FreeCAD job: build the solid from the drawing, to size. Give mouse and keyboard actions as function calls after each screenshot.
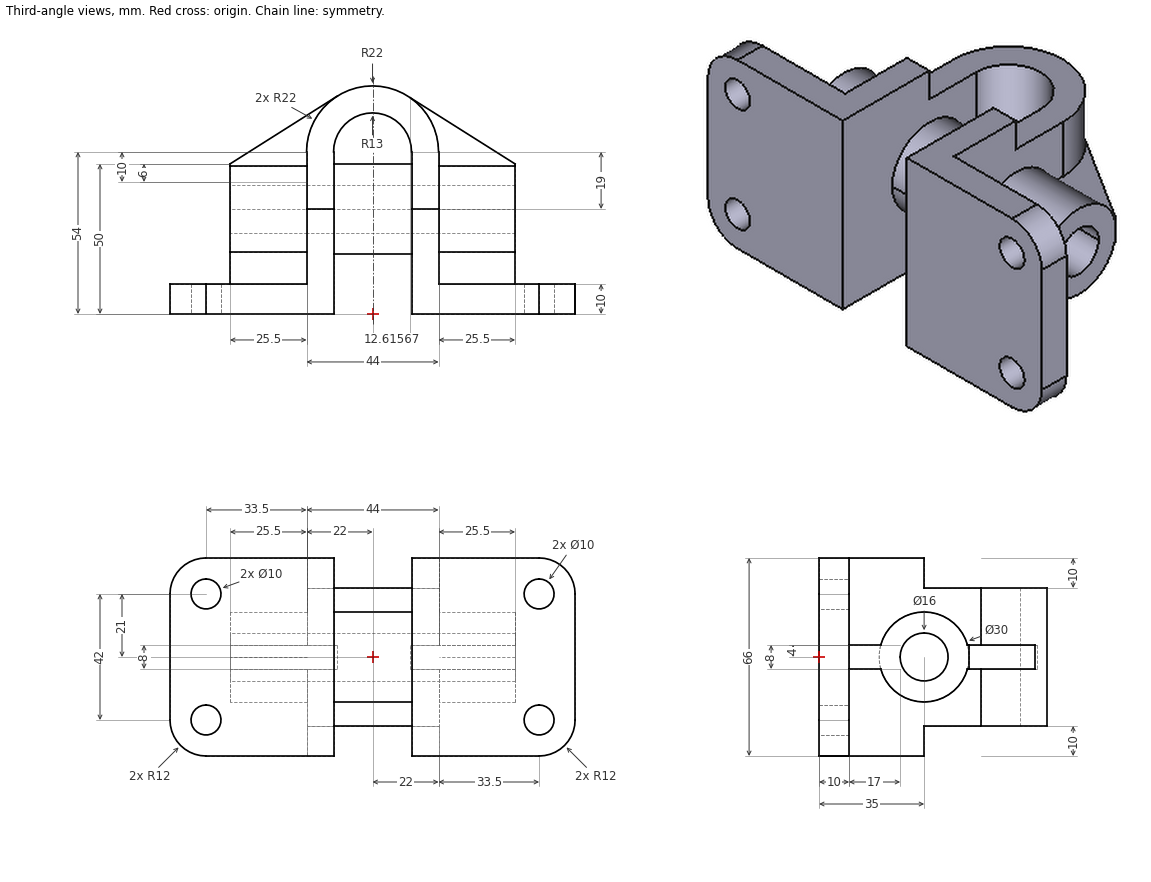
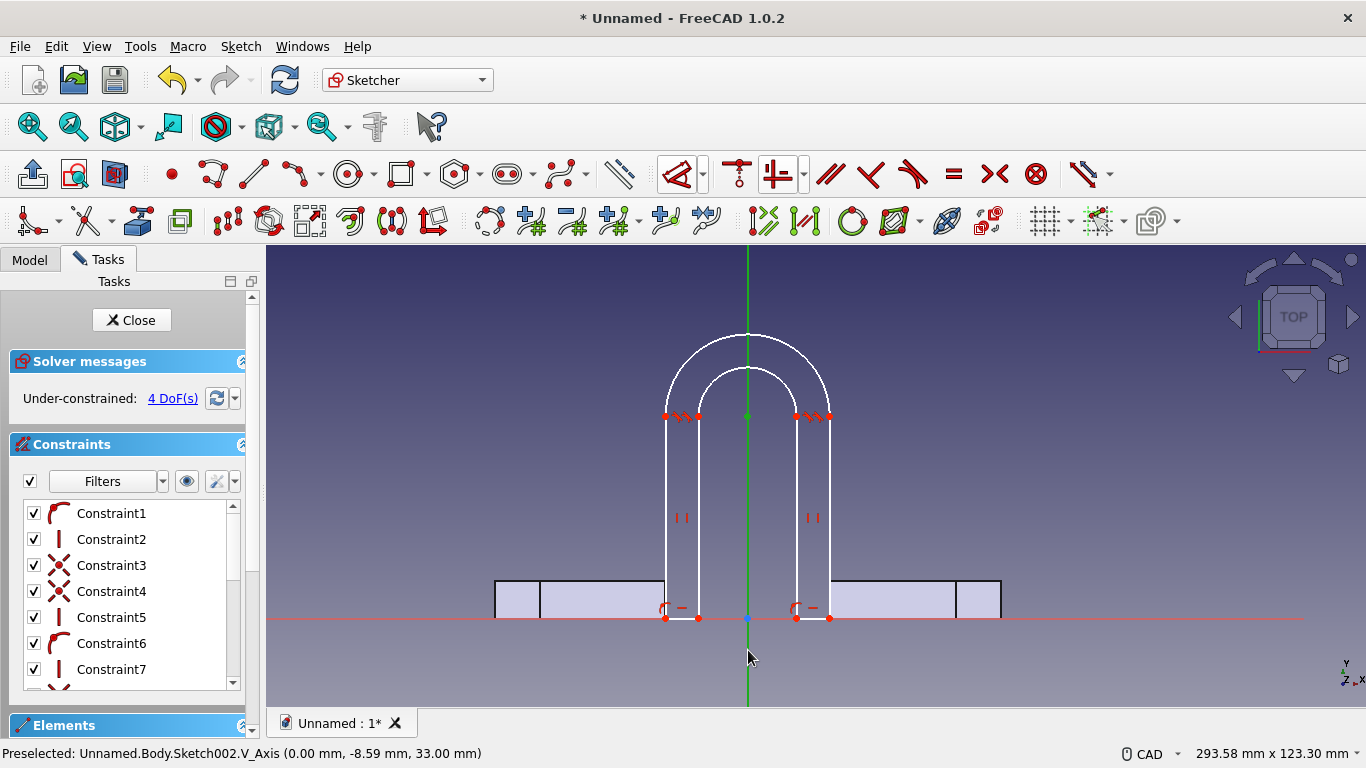
click(737, 174)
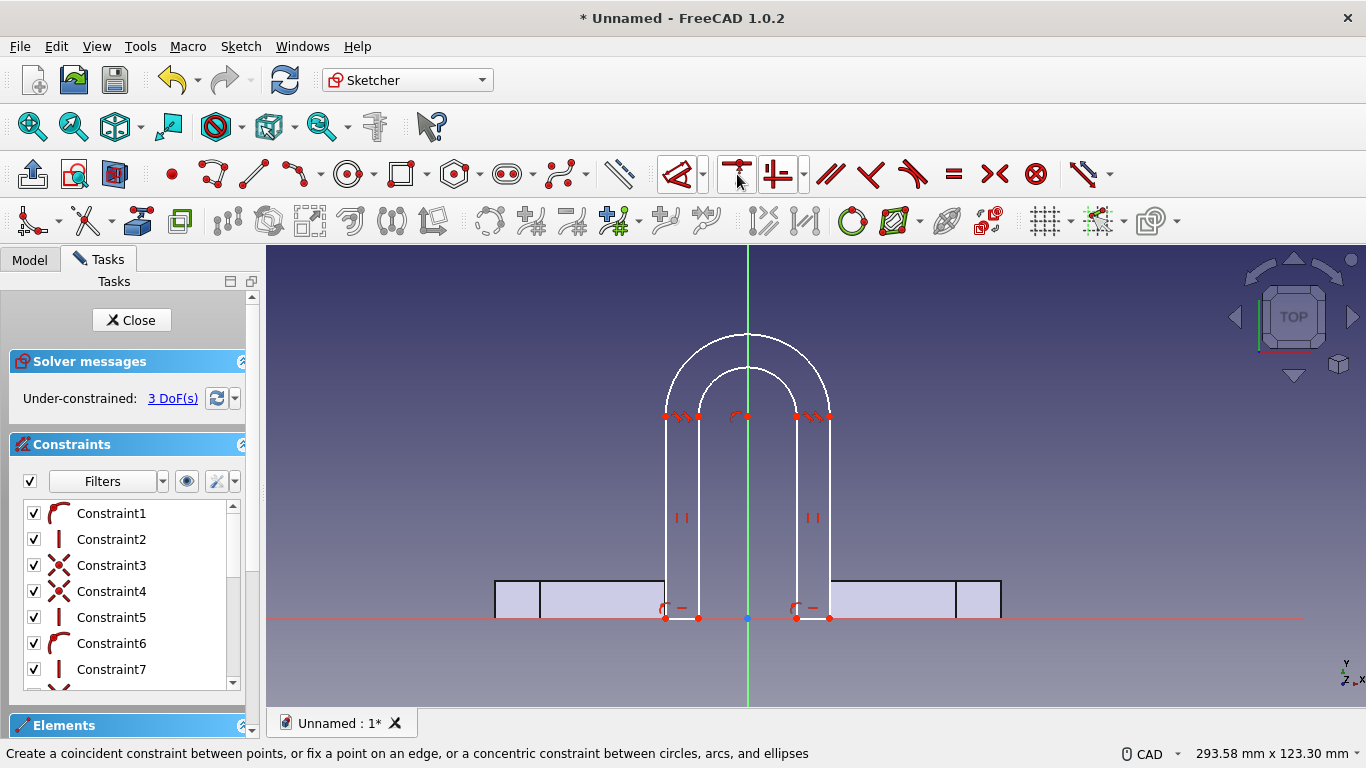
click(777, 377)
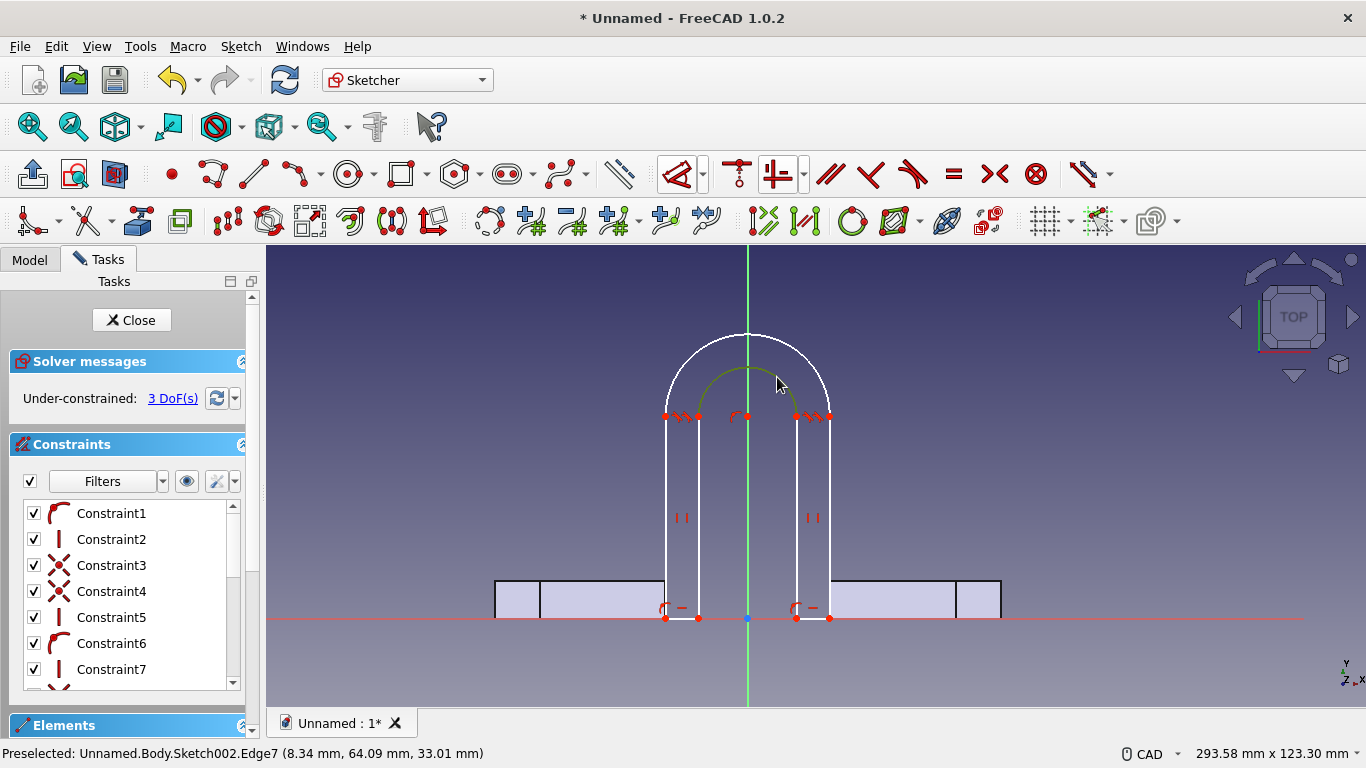
click(702, 174)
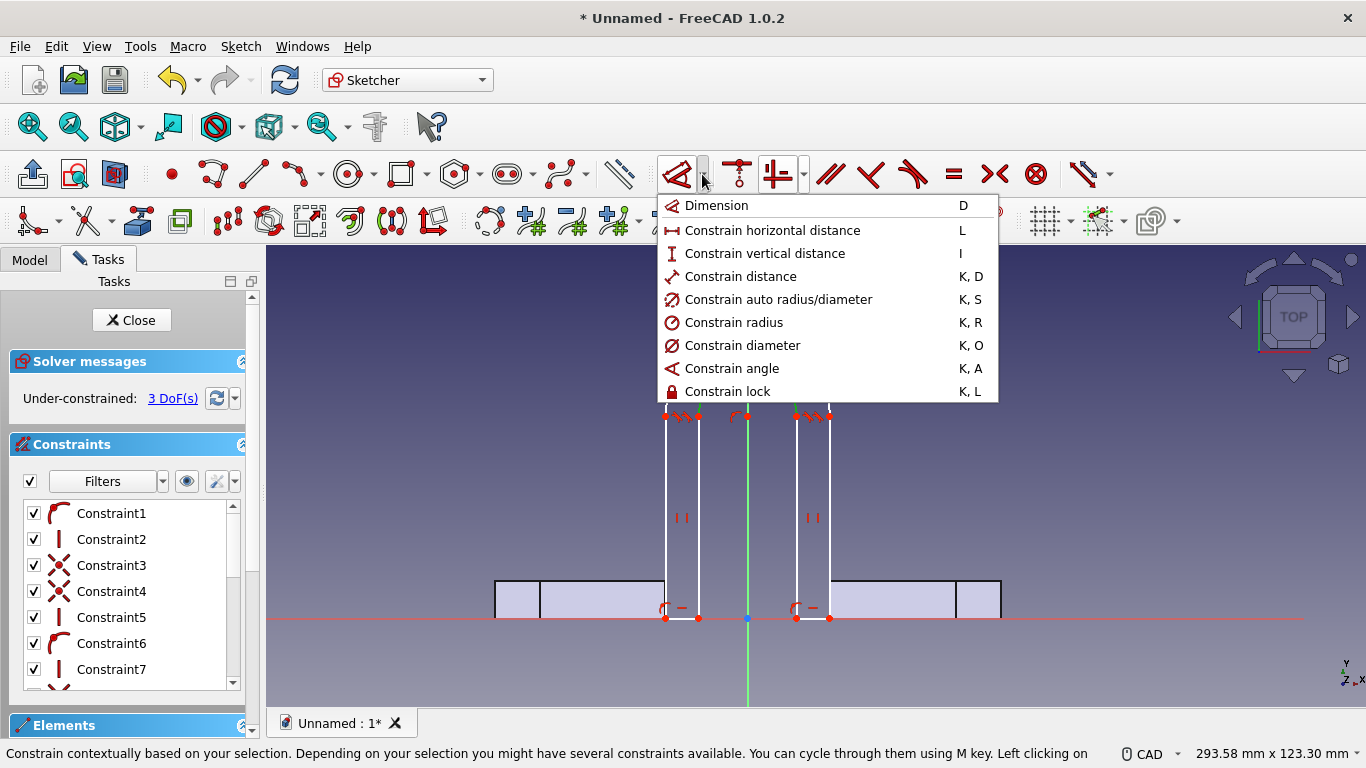
click(828, 322)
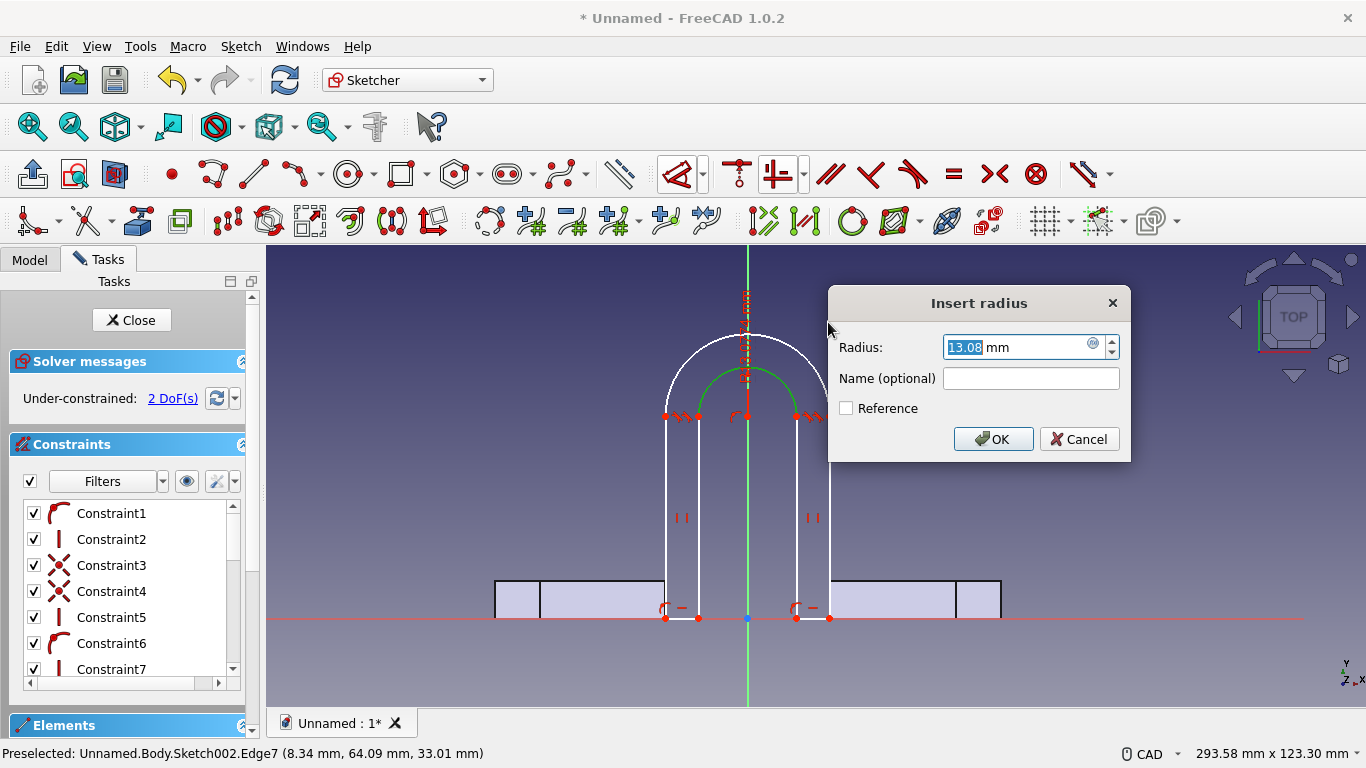
text(13)
key(Return)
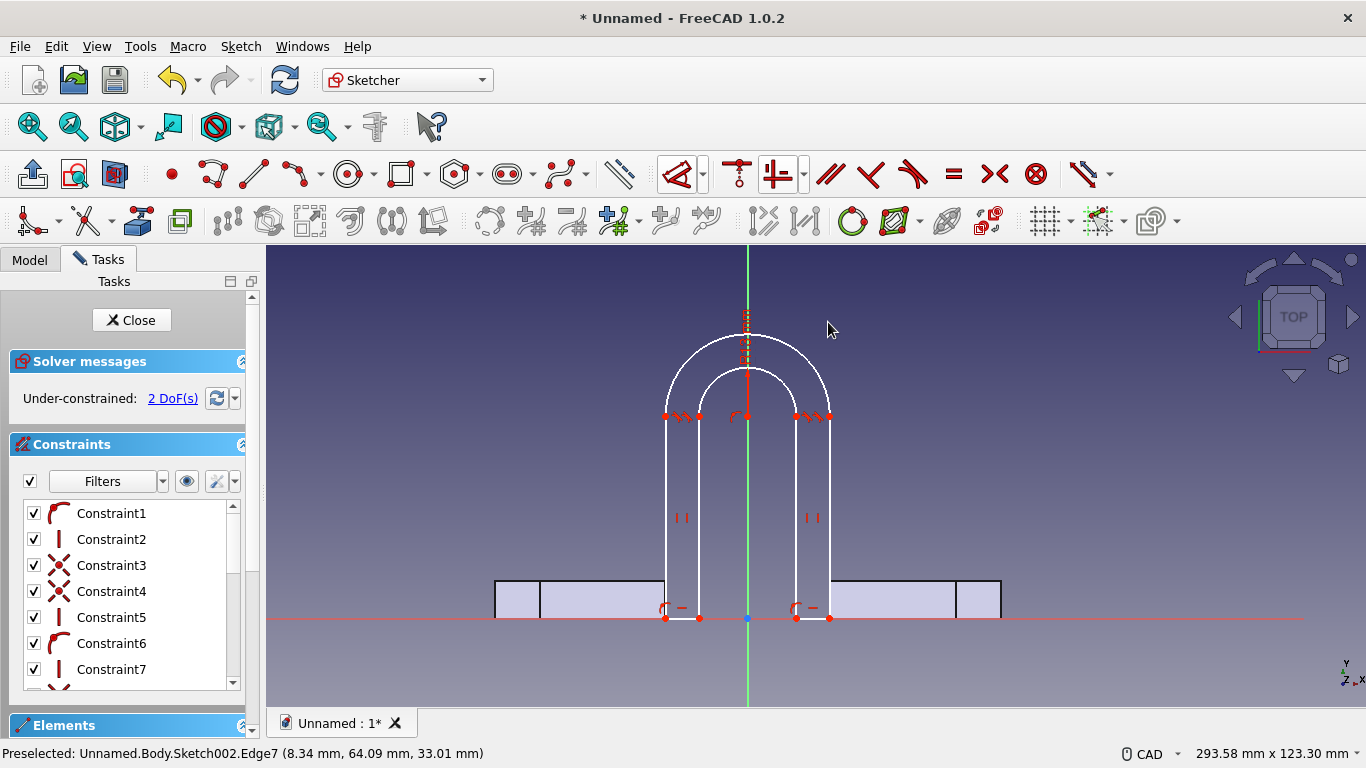
click(796, 350)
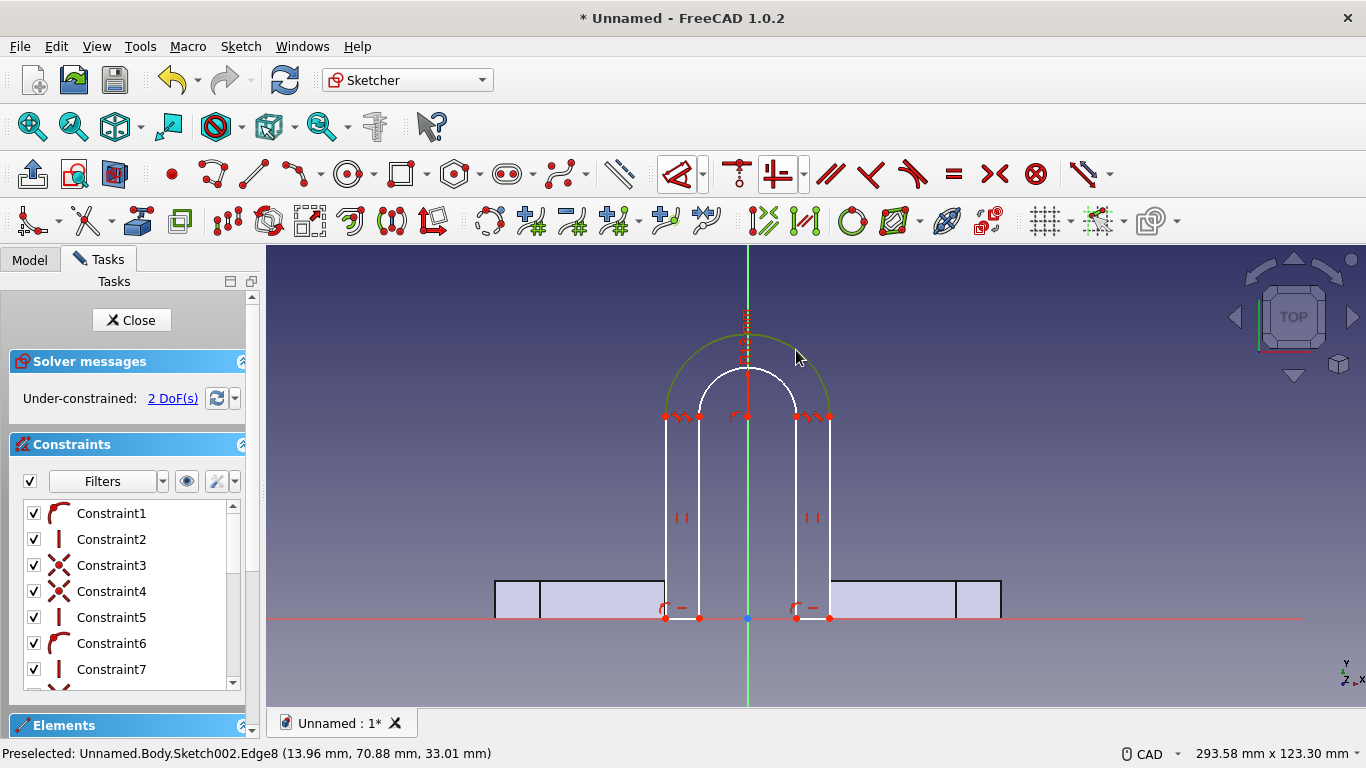
key(k)
key(r)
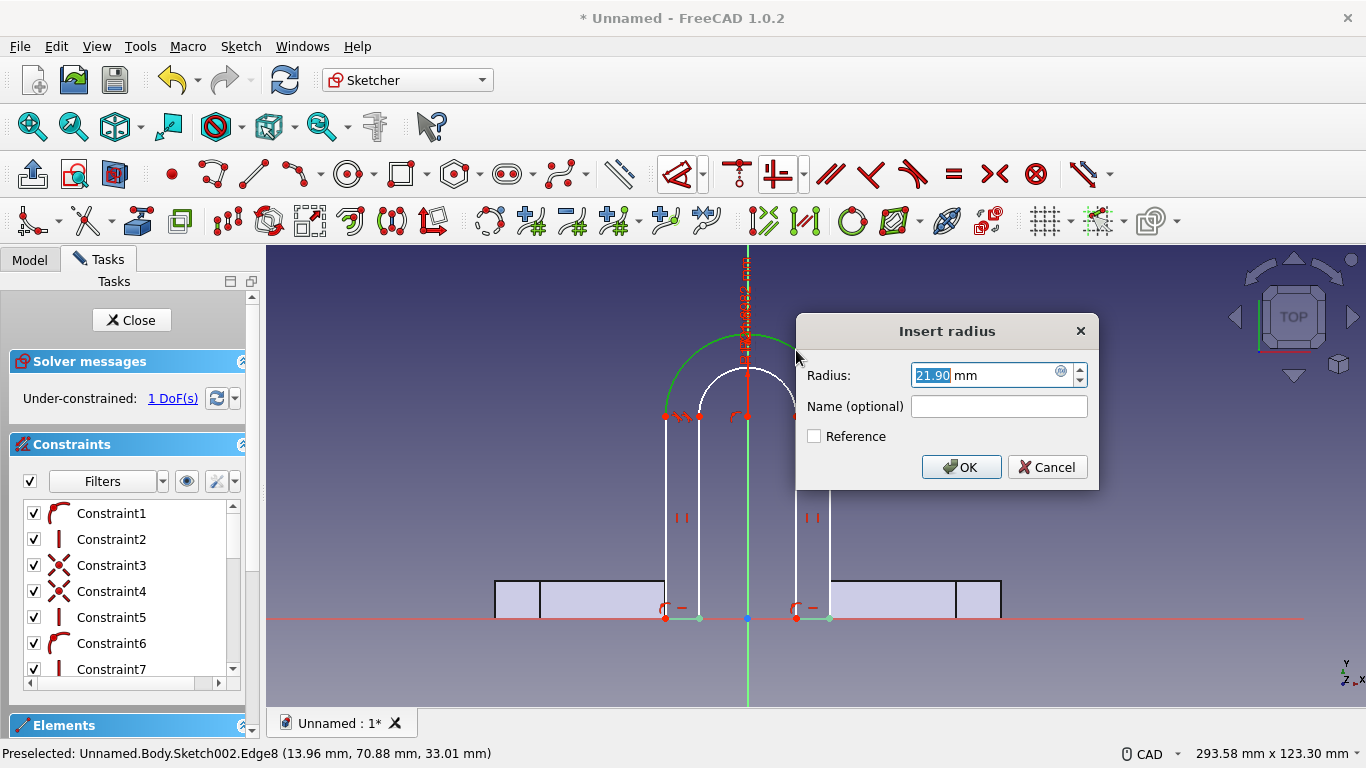
text(22)
key(Return)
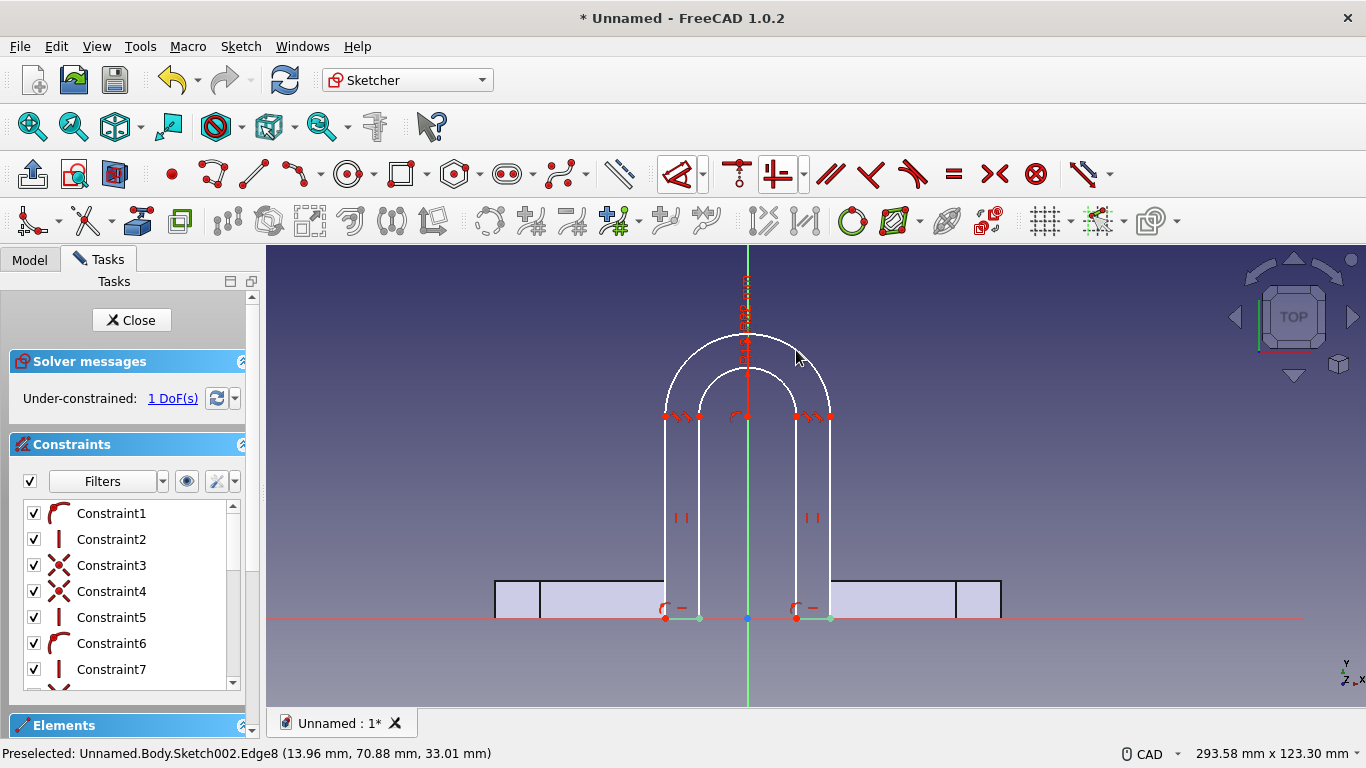
click(665, 477)